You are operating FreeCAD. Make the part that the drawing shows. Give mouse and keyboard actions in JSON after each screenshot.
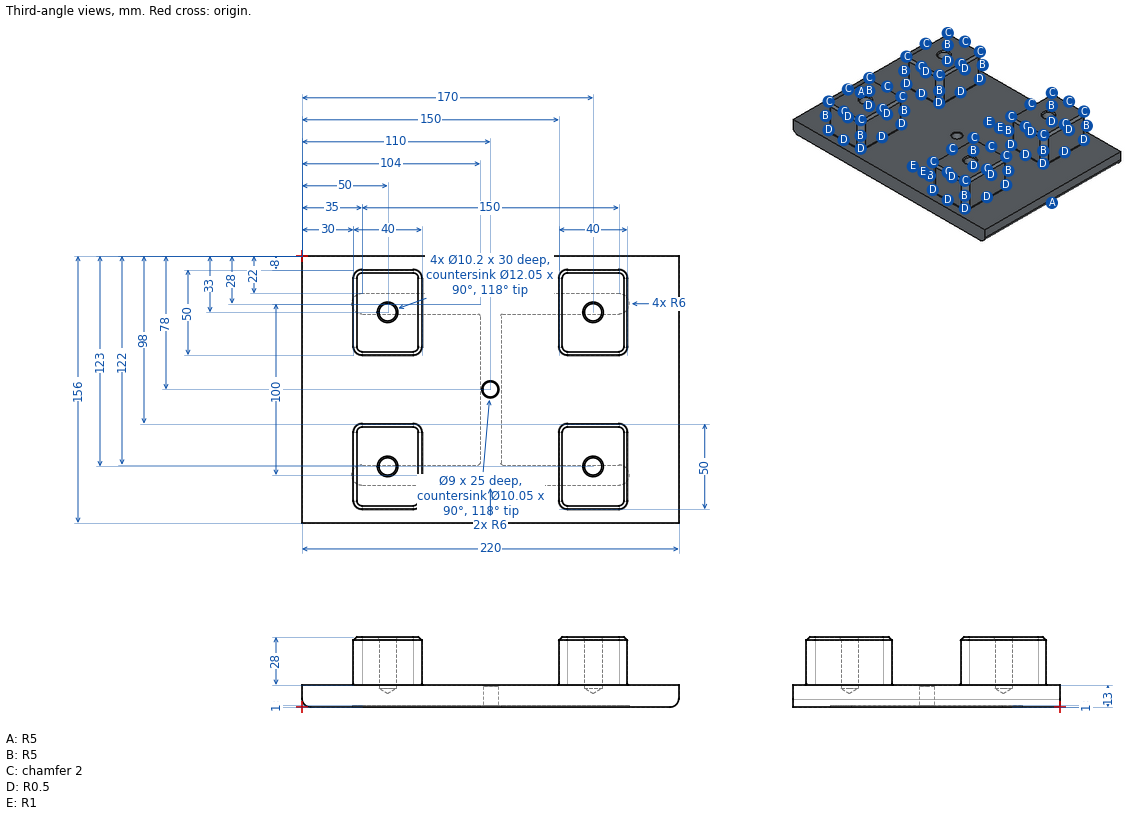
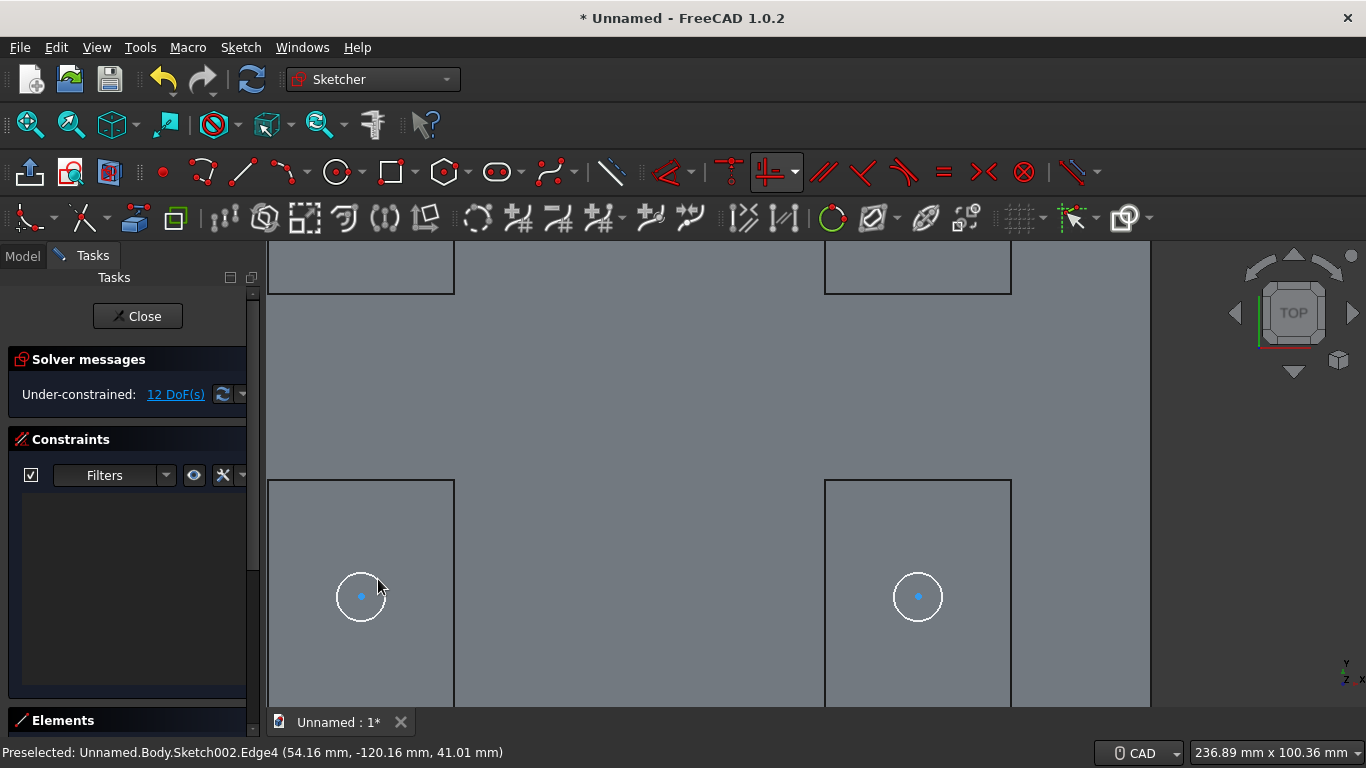
{"action": "scroll", "coordinate": [920, 598], "scroll_direction": "down", "scroll_amount": 4}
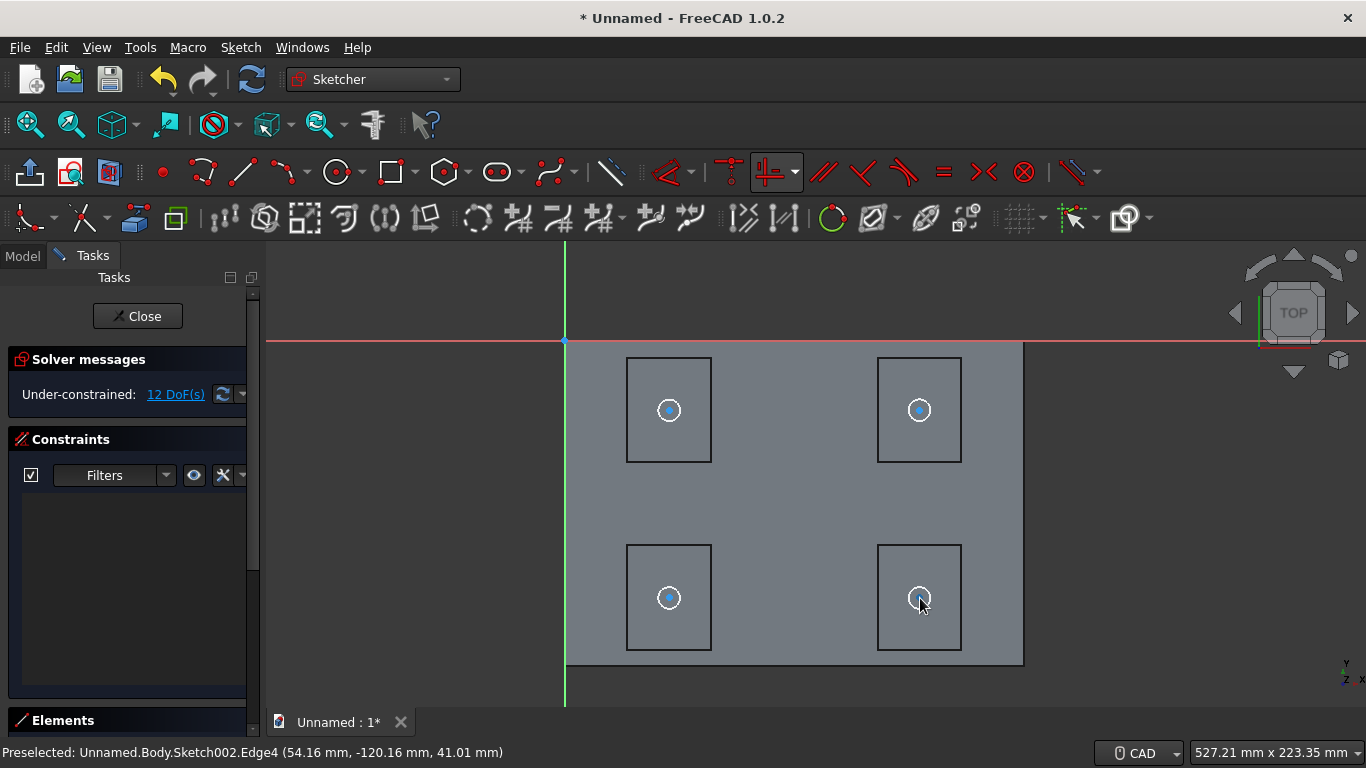
{"action": "scroll", "coordinate": [677, 403], "scroll_direction": "up", "scroll_amount": 2}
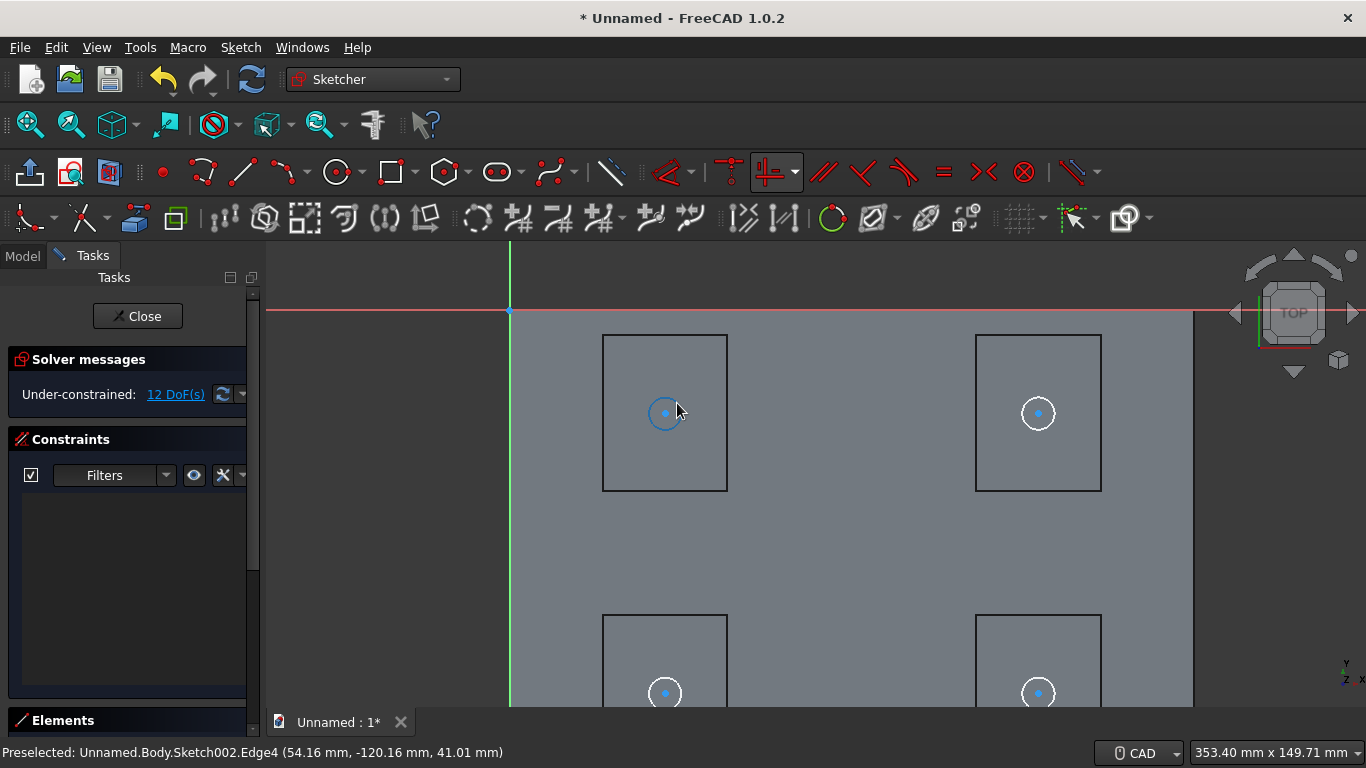
{"action": "left_click", "coordinate": [677, 402]}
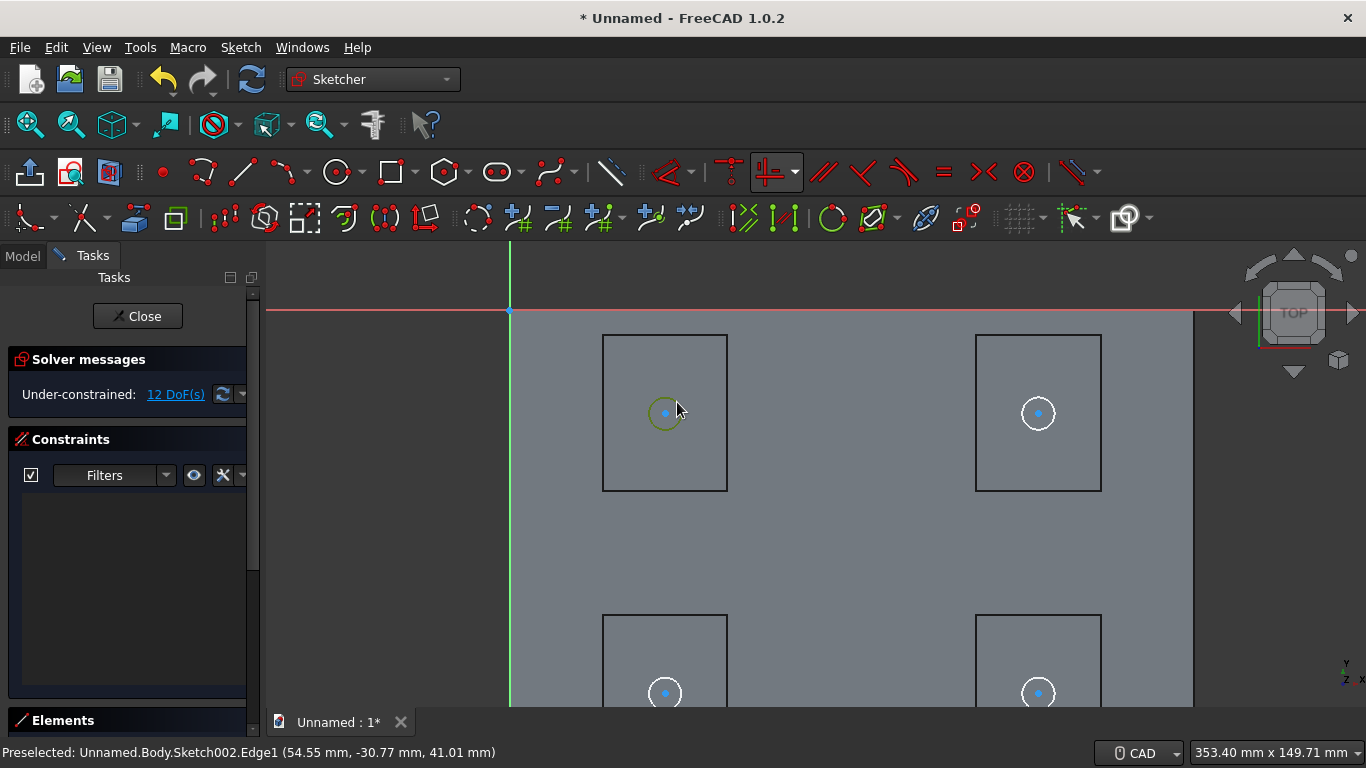
{"action": "left_click", "coordinate": [1050, 402]}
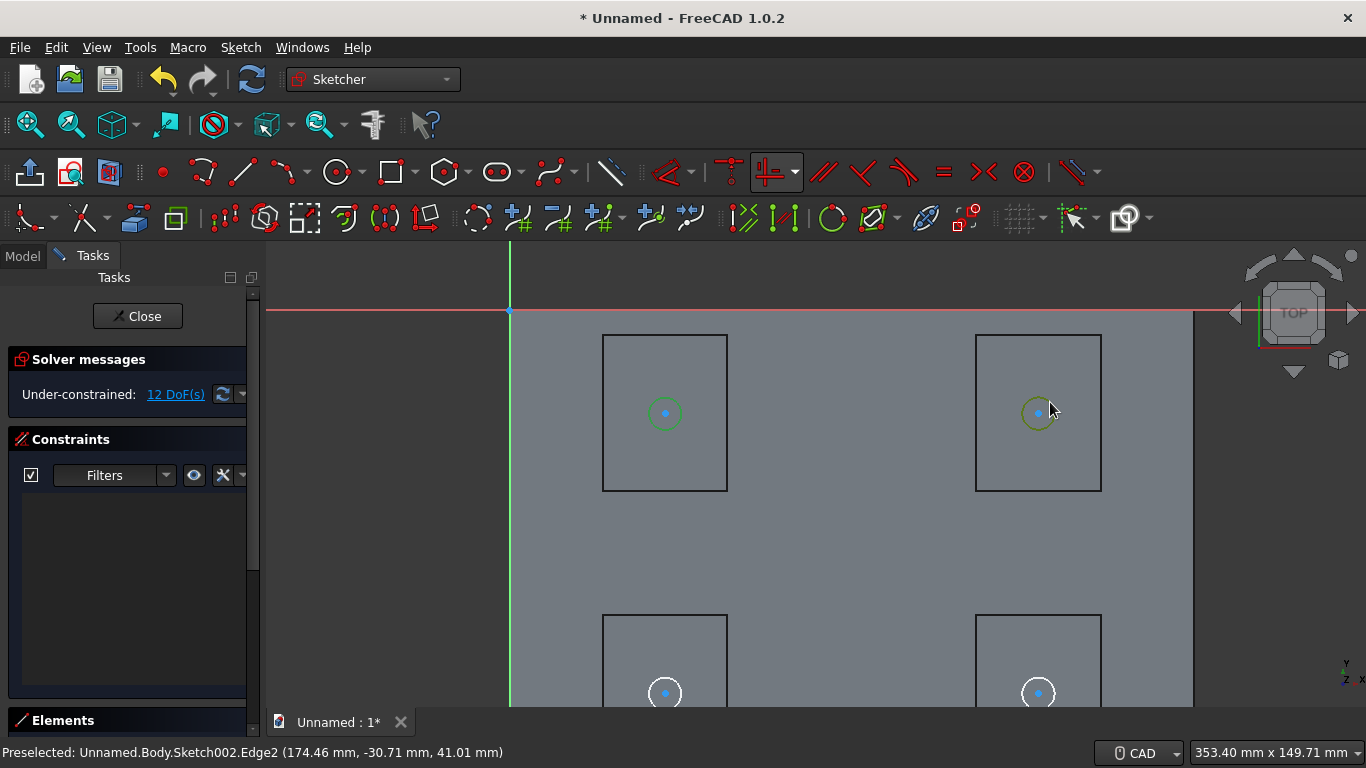
{"action": "left_click", "coordinate": [1039, 678]}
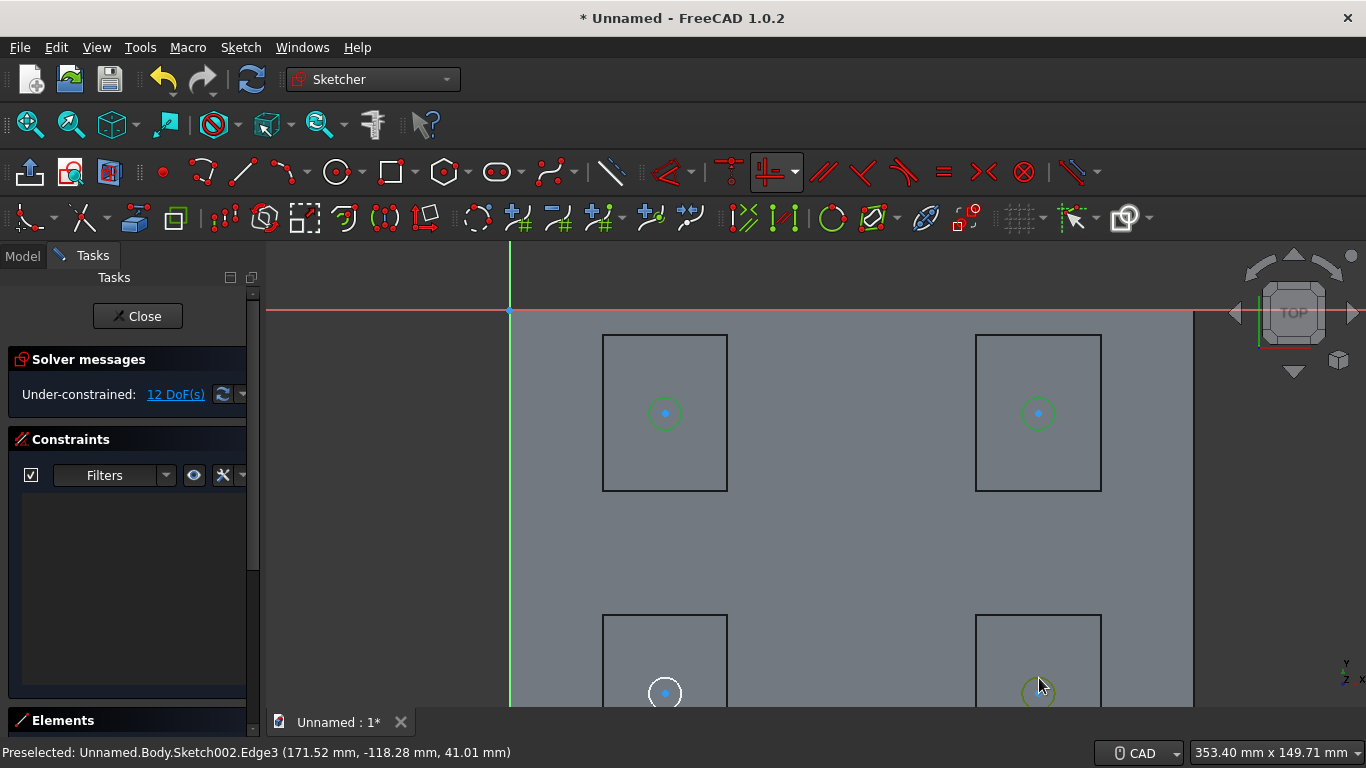
{"action": "left_click", "coordinate": [666, 678]}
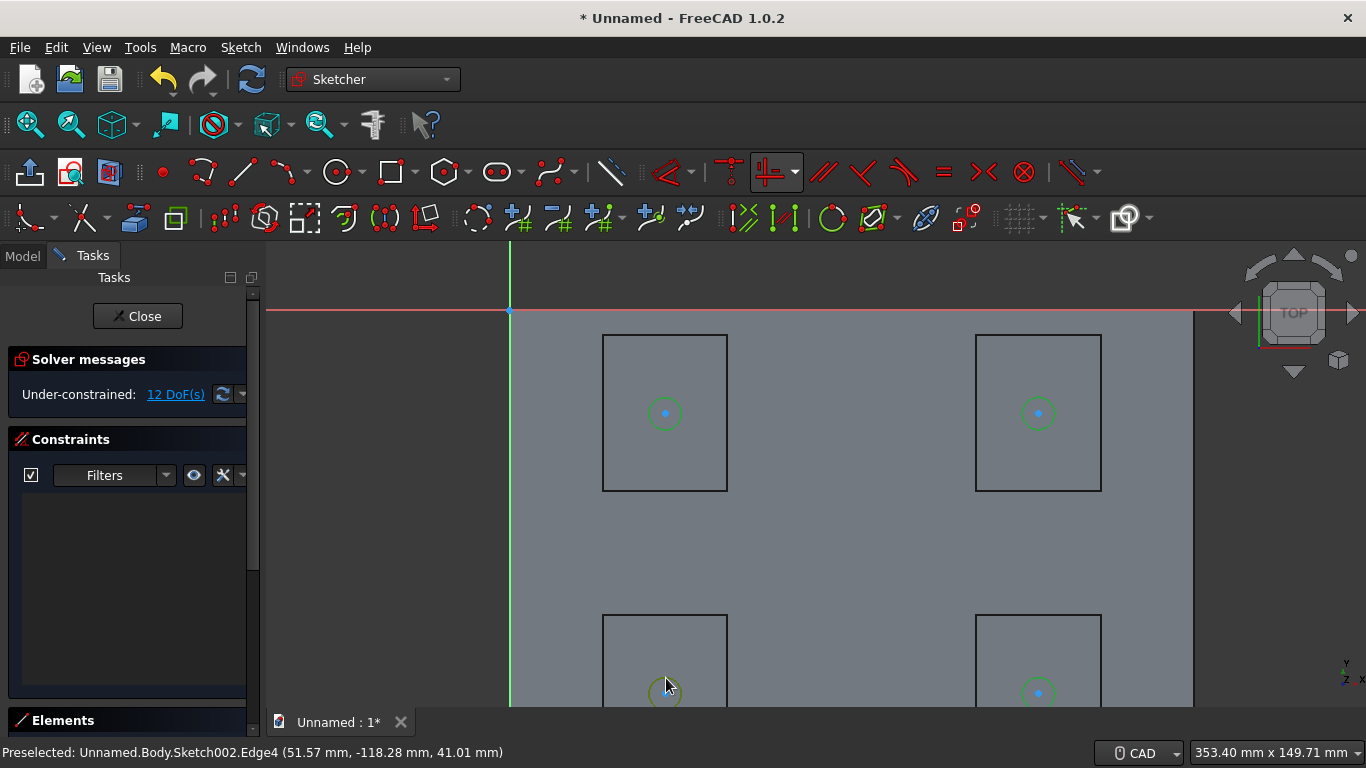
{"action": "key", "text": "e"}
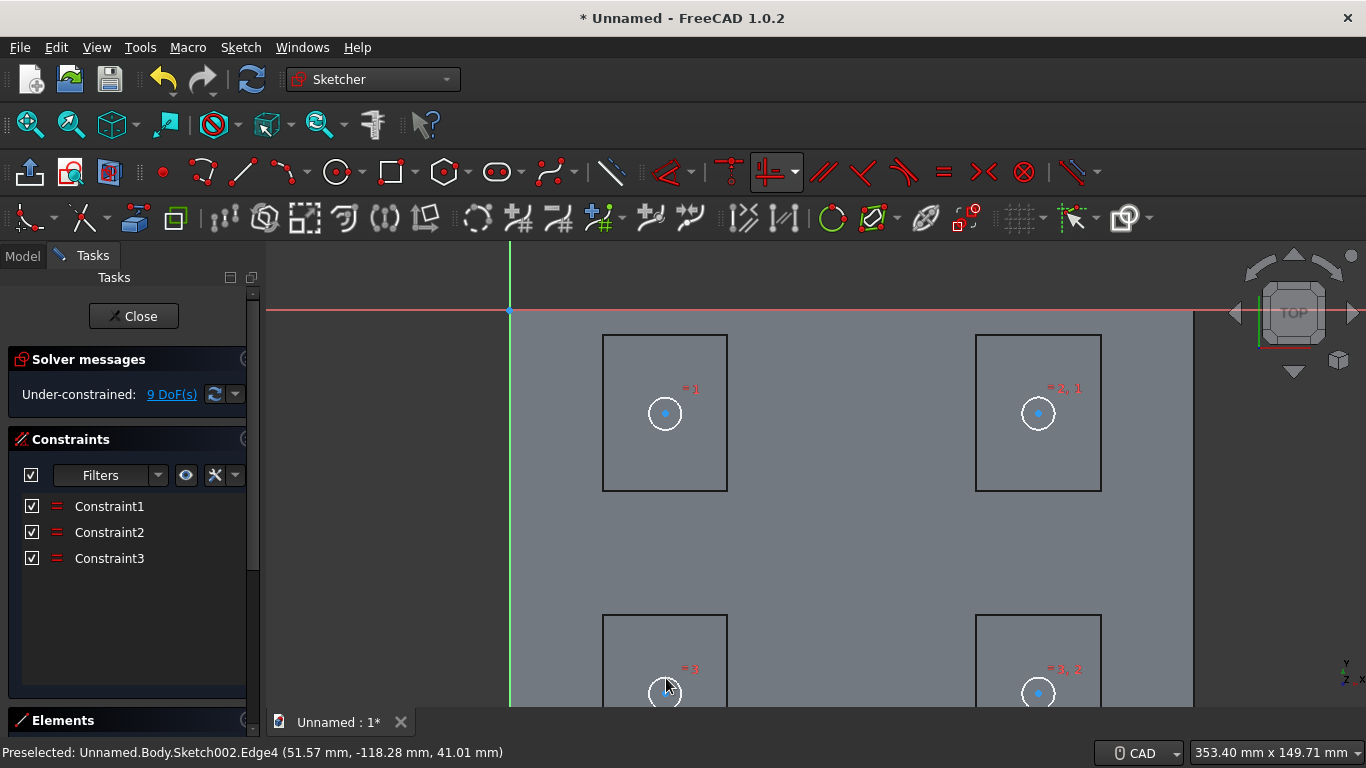
{"action": "key", "text": "d"}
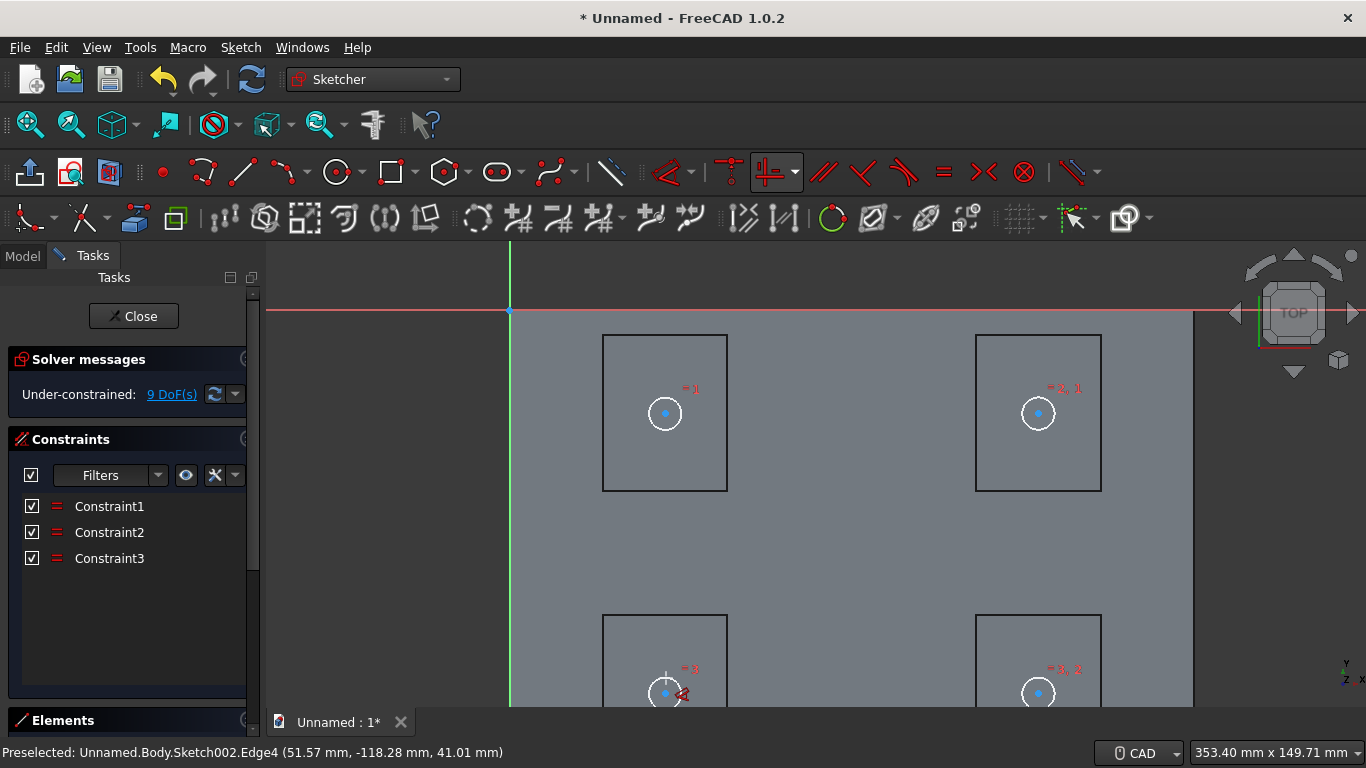
{"action": "scroll", "coordinate": [677, 402], "scroll_direction": "up", "scroll_amount": 2}